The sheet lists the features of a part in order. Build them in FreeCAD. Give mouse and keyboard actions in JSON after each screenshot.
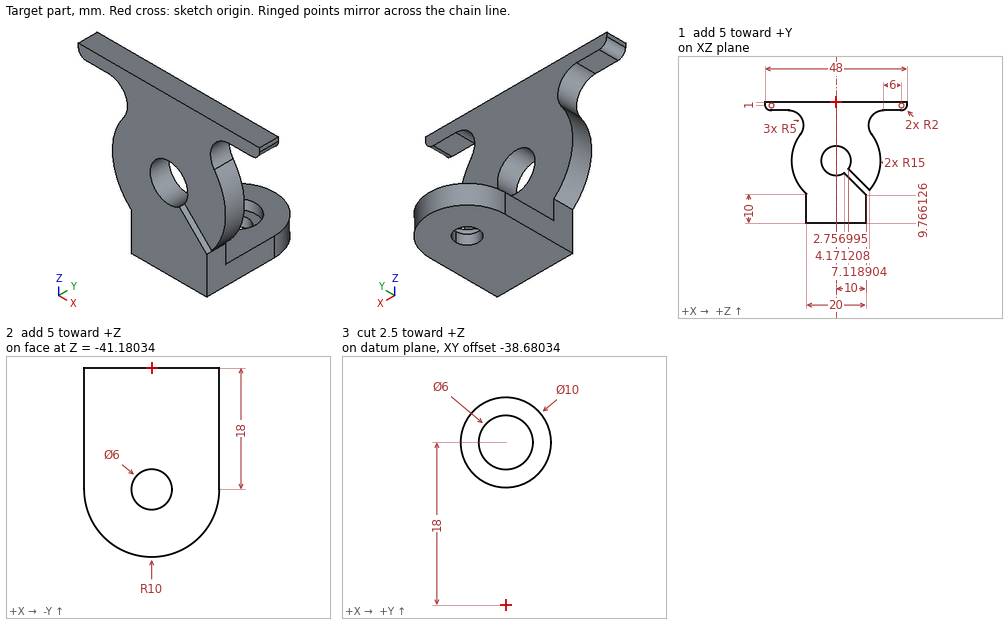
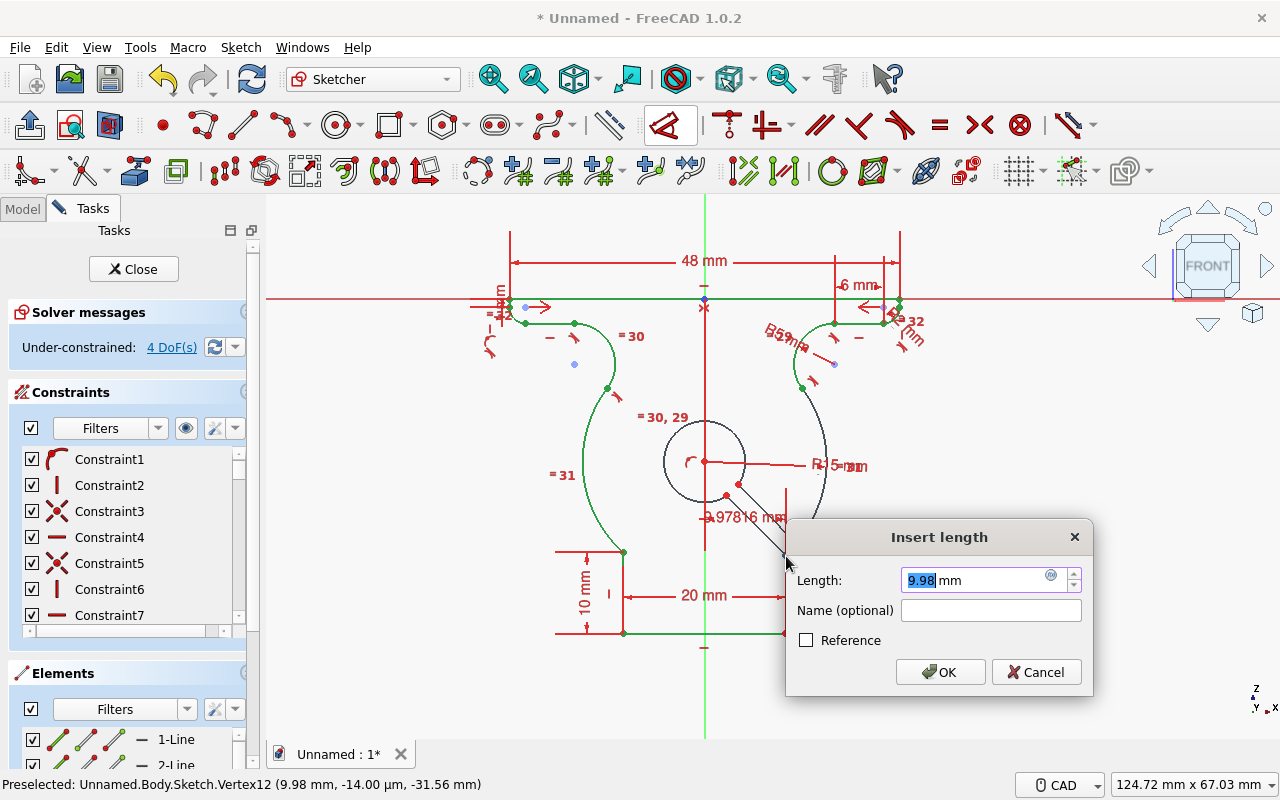
{"action": "type", "text": "10"}
{"action": "key", "text": "Return"}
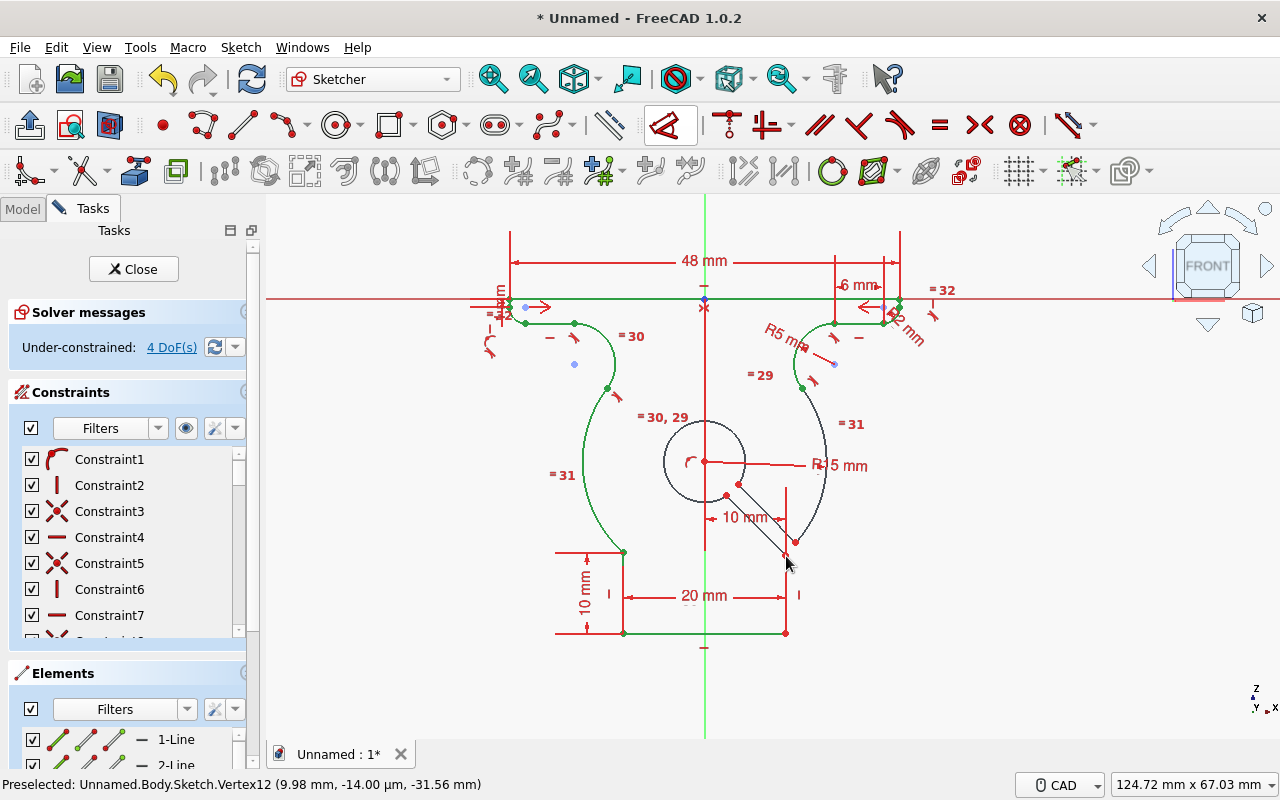
{"action": "left_click", "coordinate": [786, 579]}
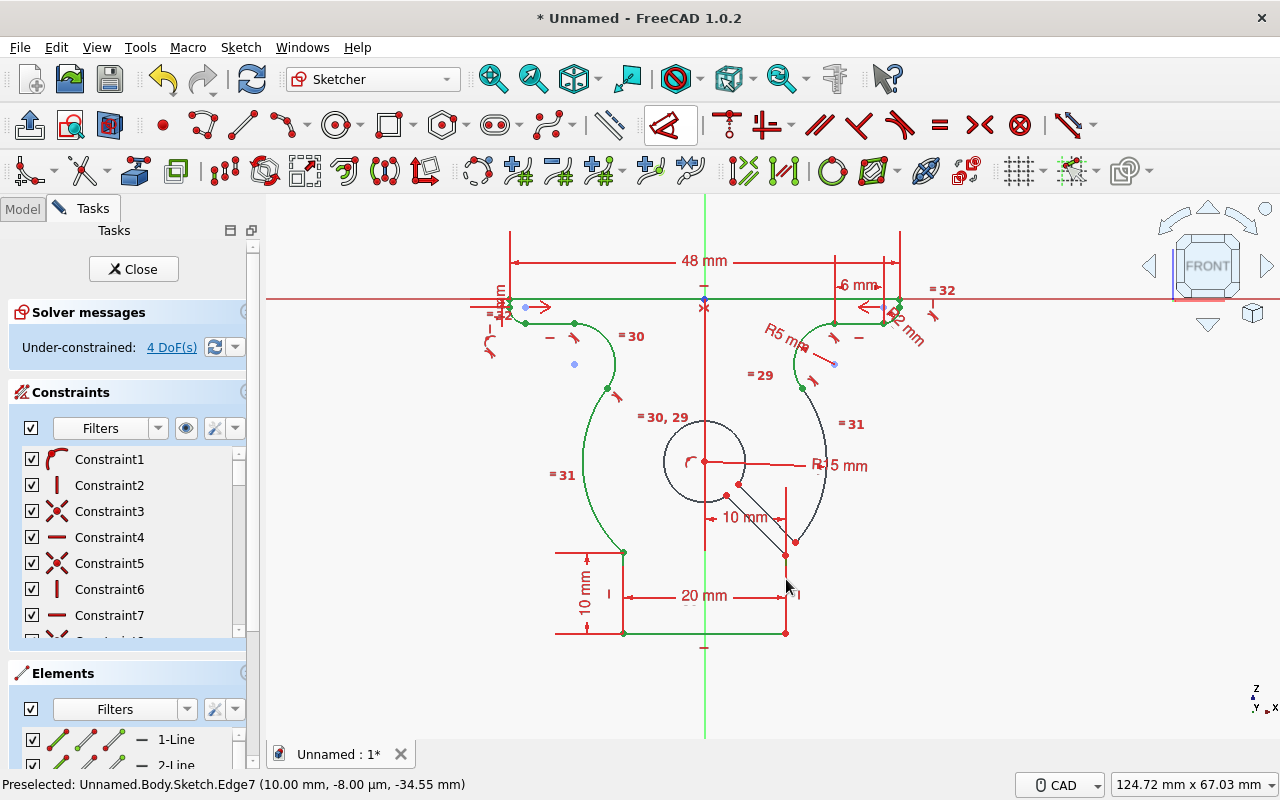
{"action": "key", "text": "i"}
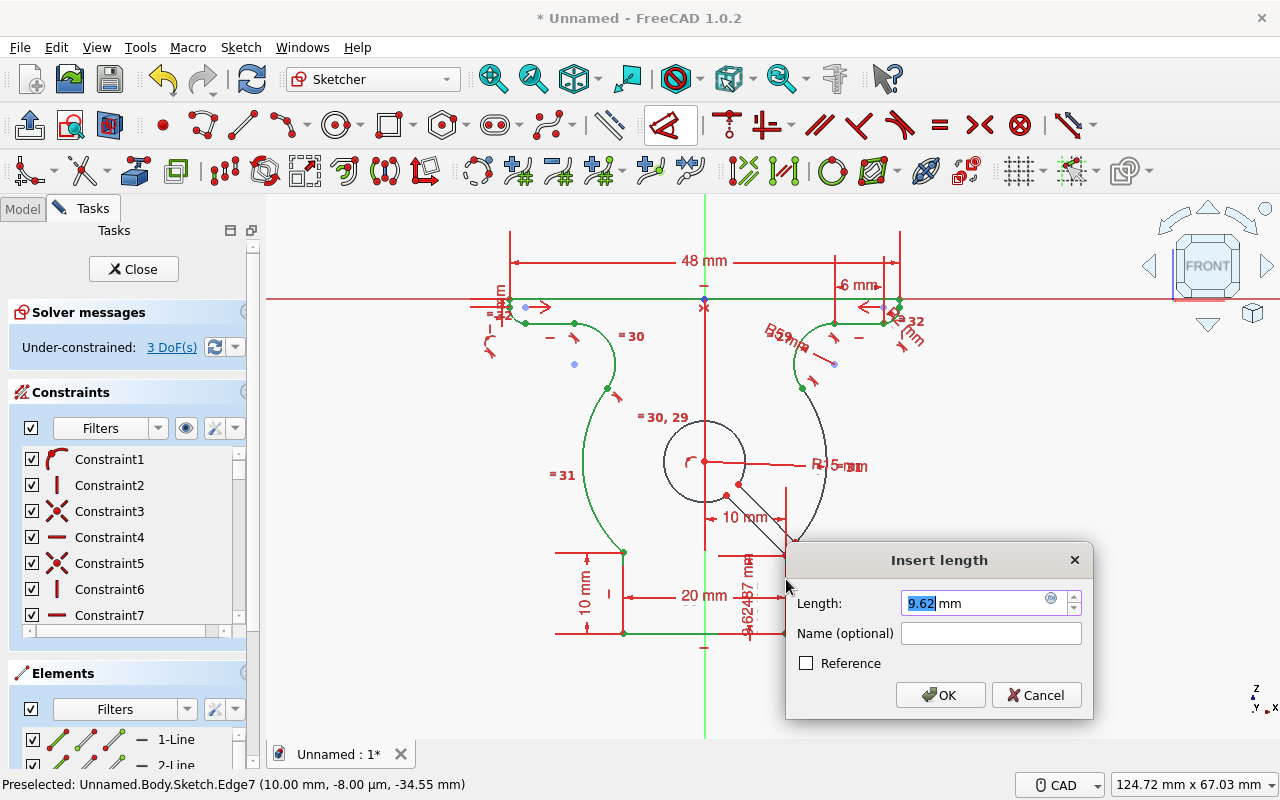
{"action": "type", "text": "9.766126"}
{"action": "key", "text": "Return"}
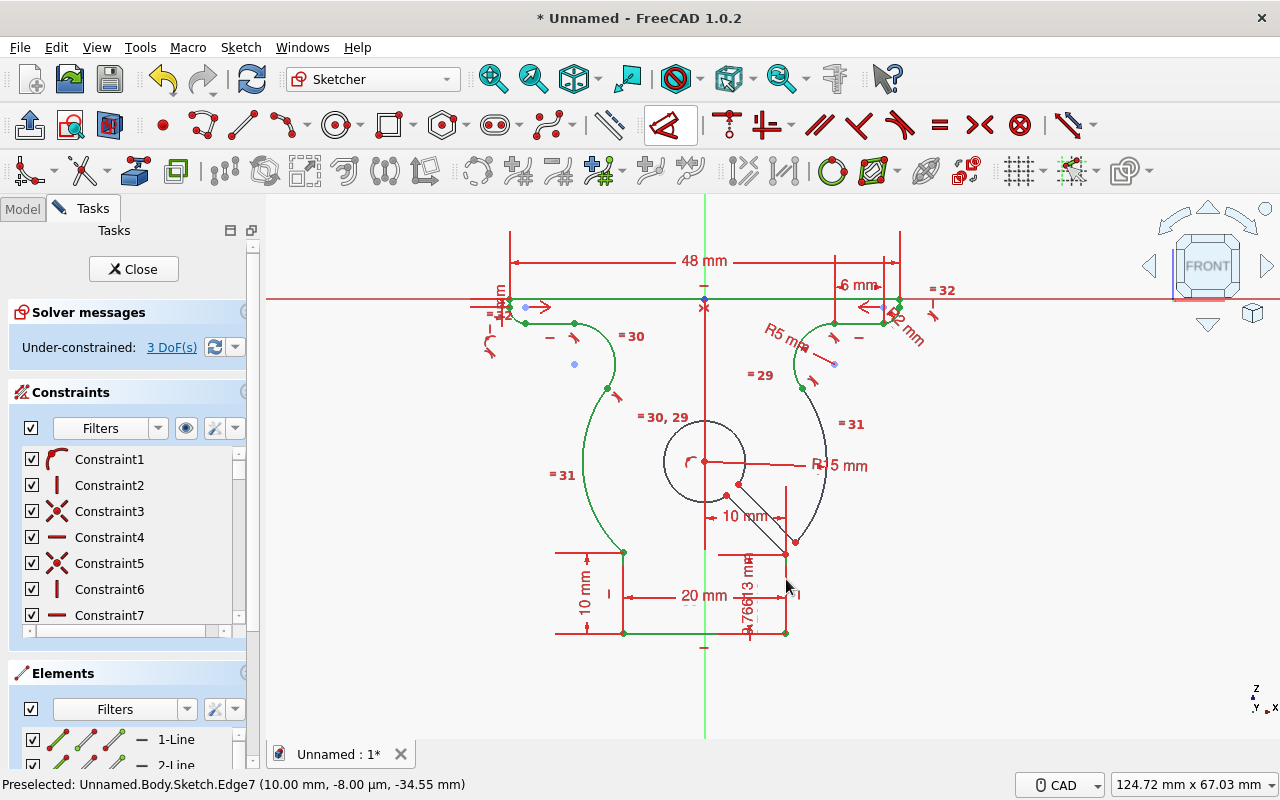
{"action": "left_click", "coordinate": [738, 485]}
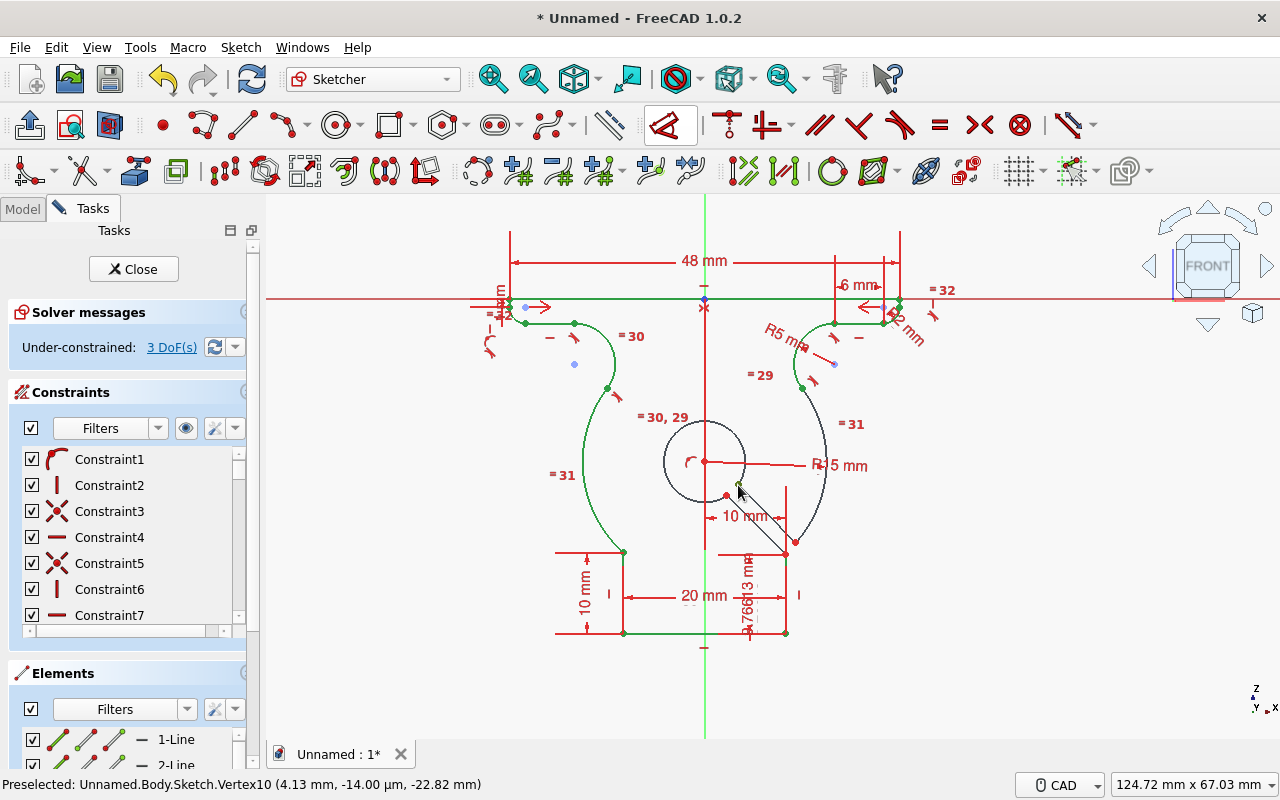
{"action": "key", "text": "l"}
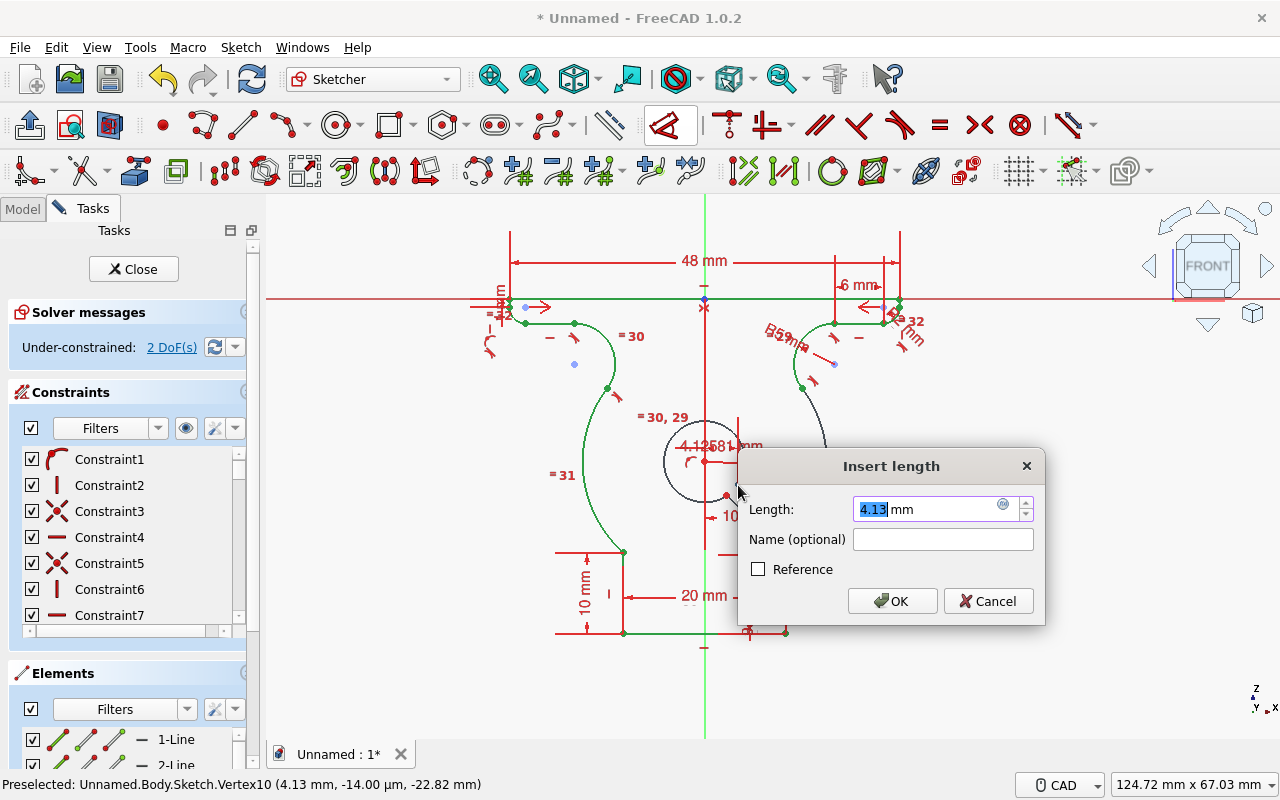
{"action": "type", "text": "4.171208"}
{"action": "key", "text": "Return"}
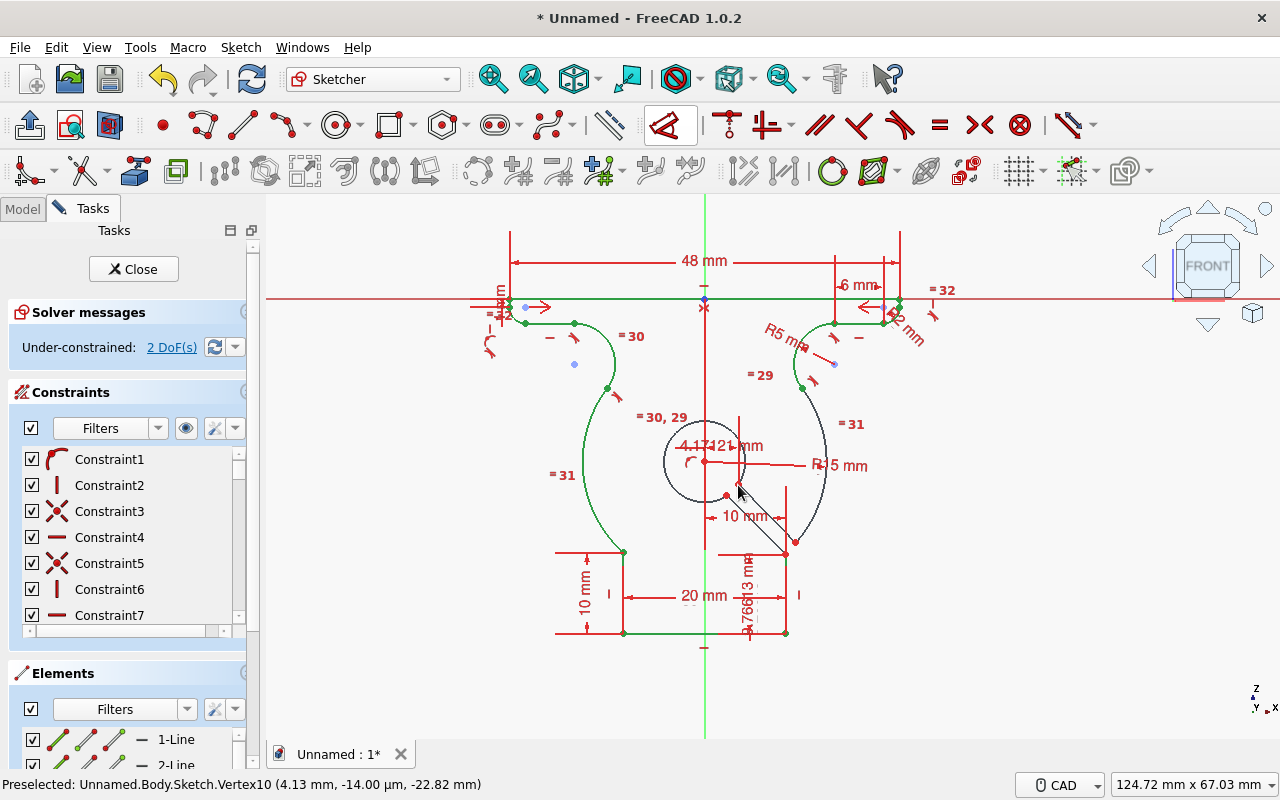
{"action": "scroll", "coordinate": [727, 496], "scroll_direction": "up", "scroll_amount": 3}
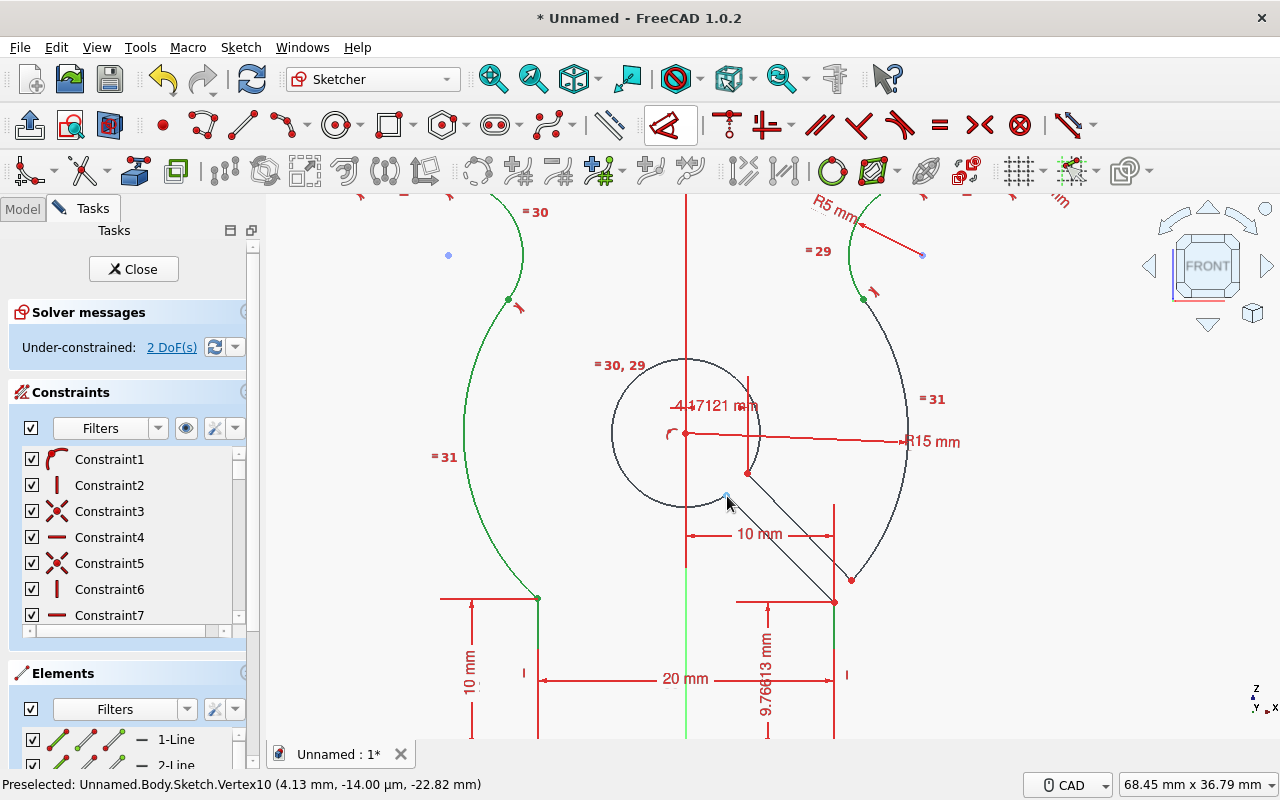
{"action": "left_click", "coordinate": [726, 495]}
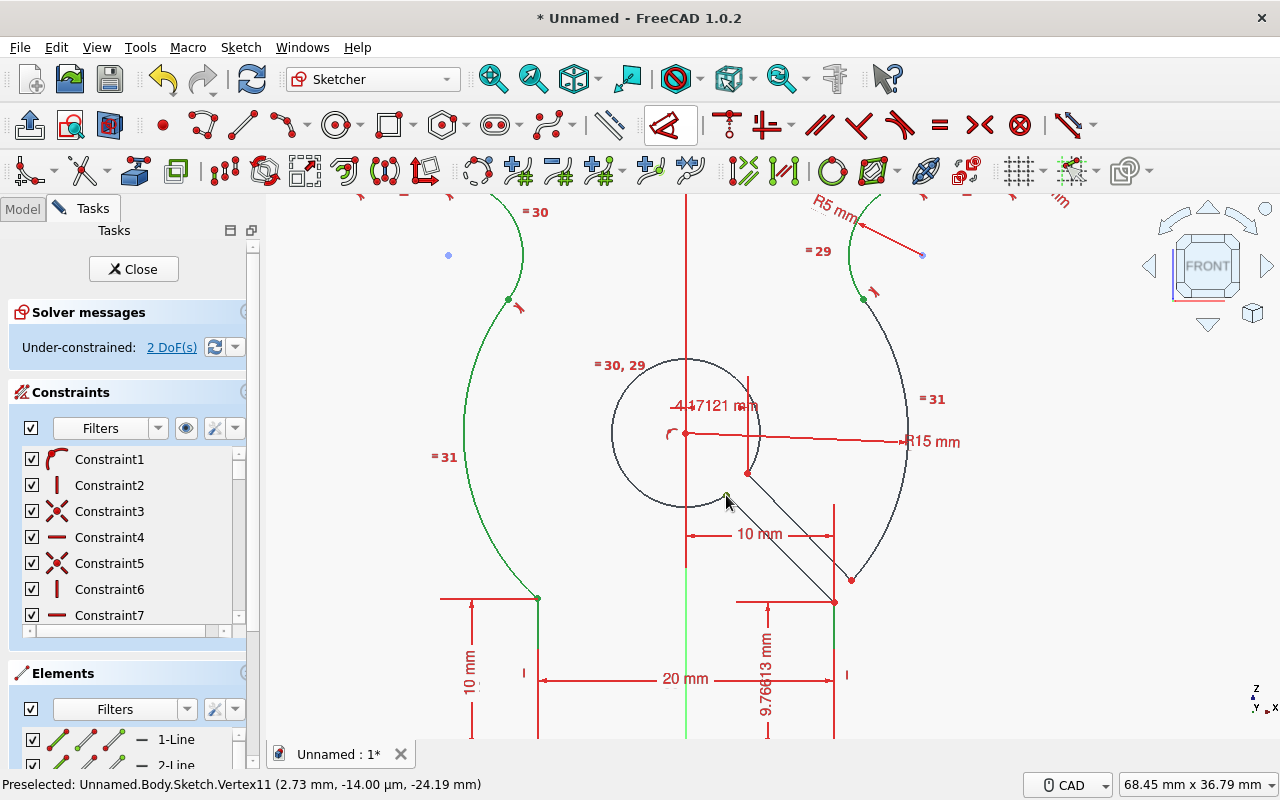
{"action": "key", "text": "l"}